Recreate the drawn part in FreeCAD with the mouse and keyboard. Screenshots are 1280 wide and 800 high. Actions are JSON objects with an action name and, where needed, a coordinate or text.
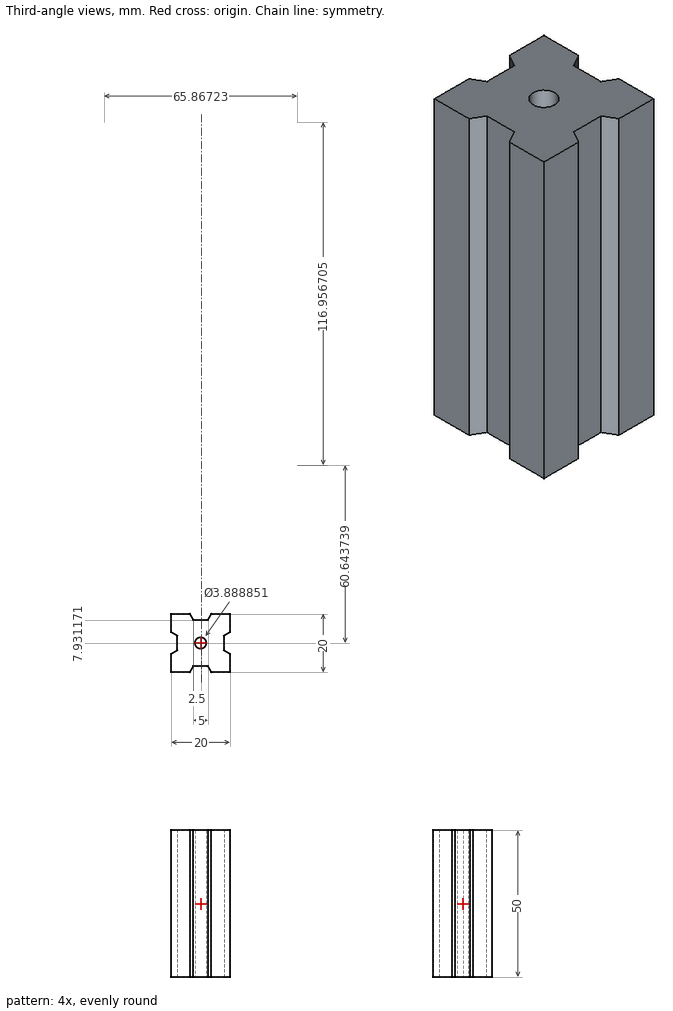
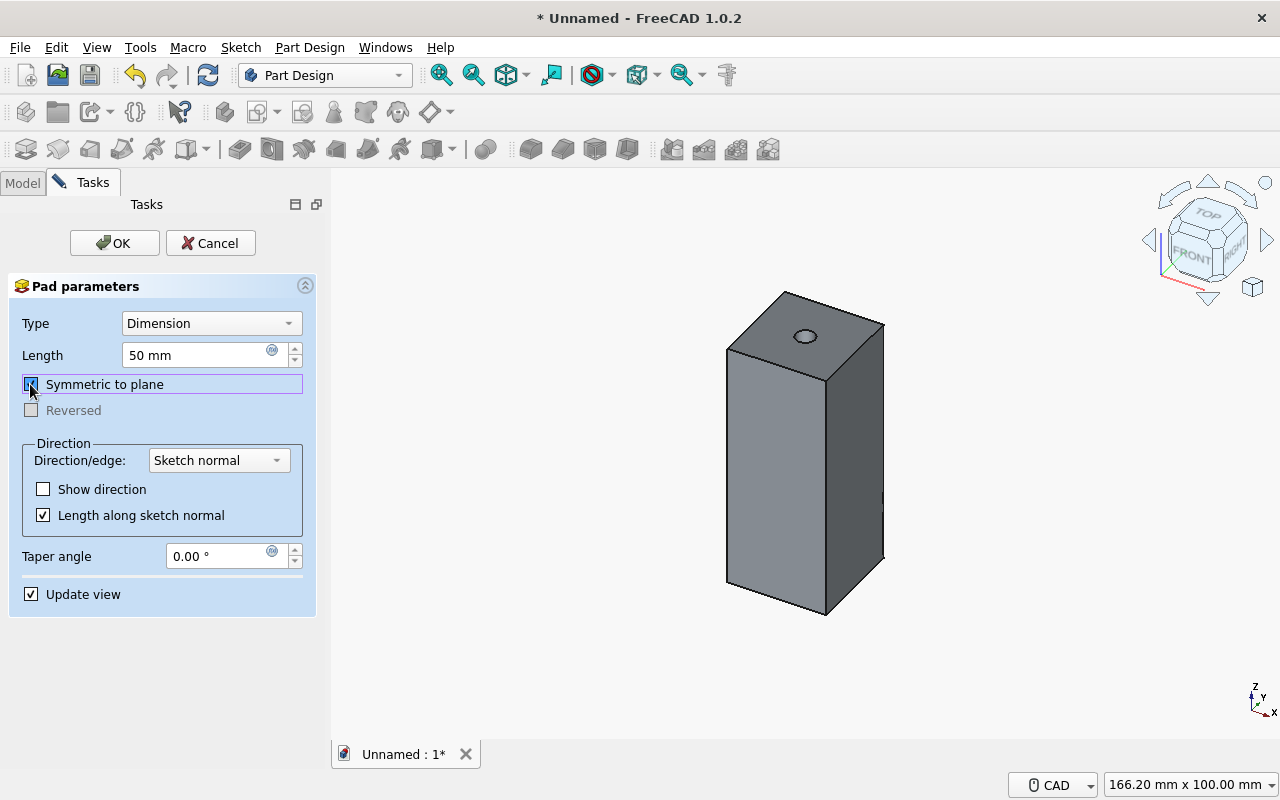
{"action": "left_click", "coordinate": [115, 243]}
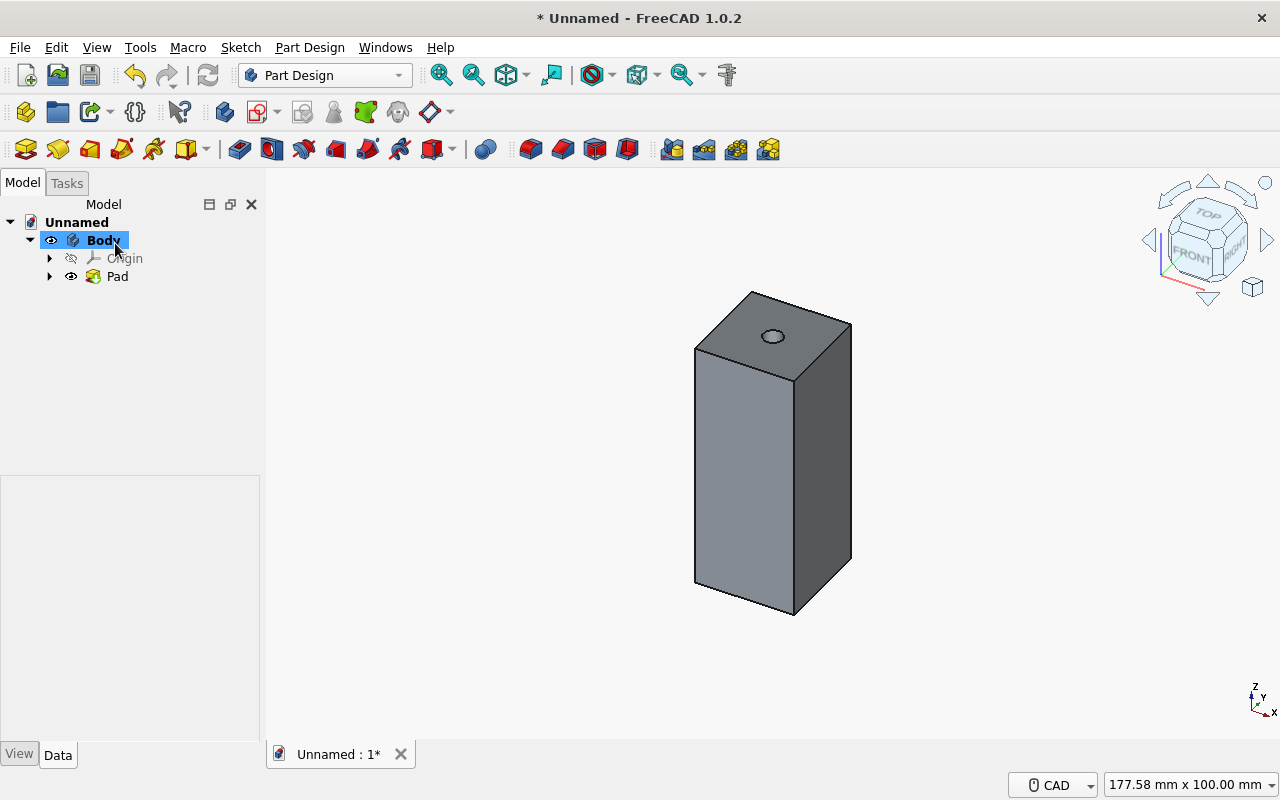
{"action": "left_click", "coordinate": [818, 329]}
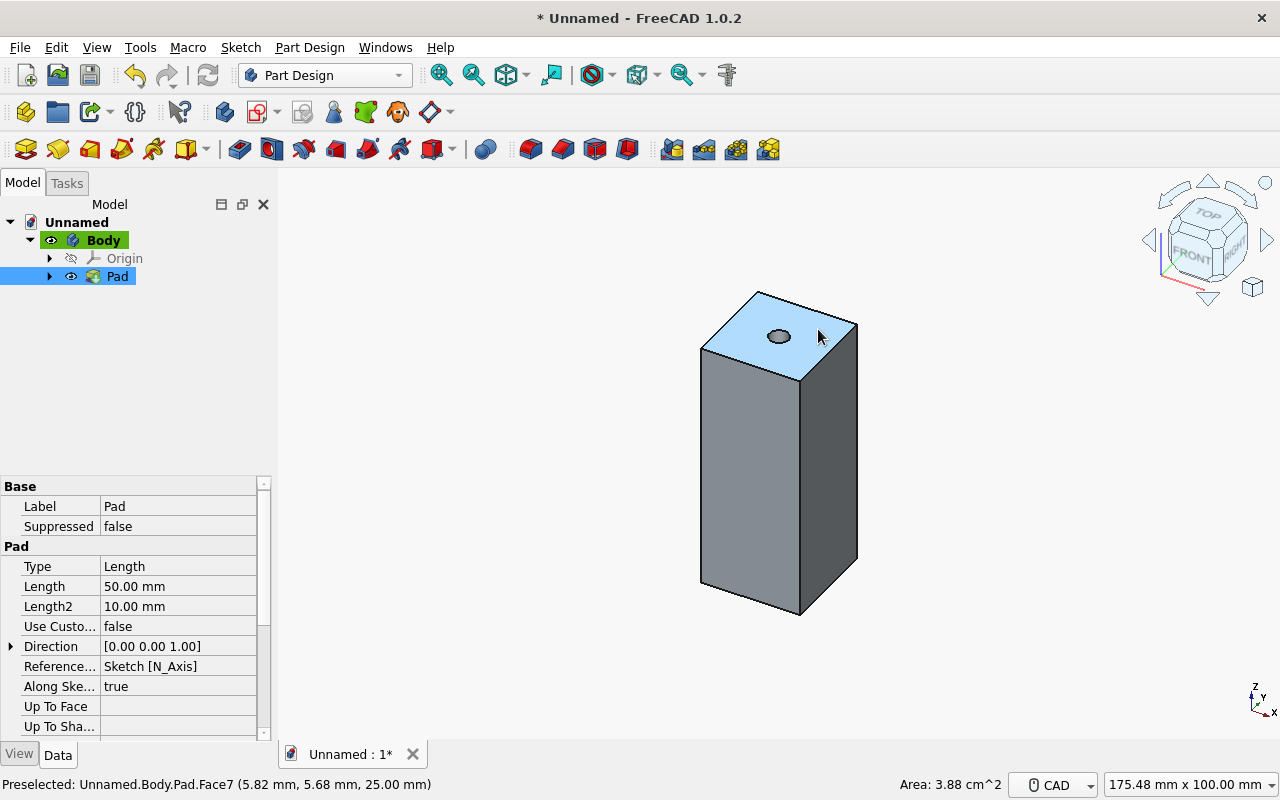
{"action": "left_click", "coordinate": [258, 112]}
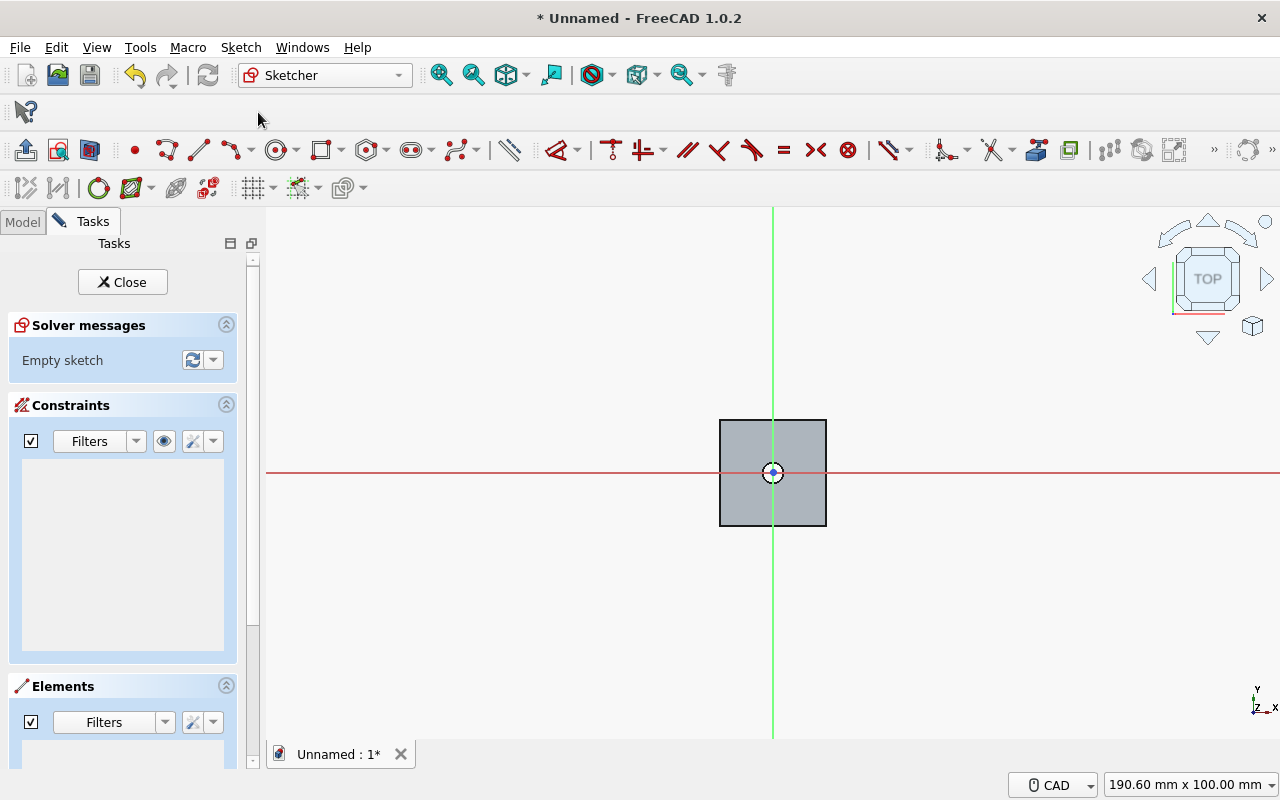
{"action": "scroll", "coordinate": [665, 711], "scroll_direction": "down", "scroll_amount": 5}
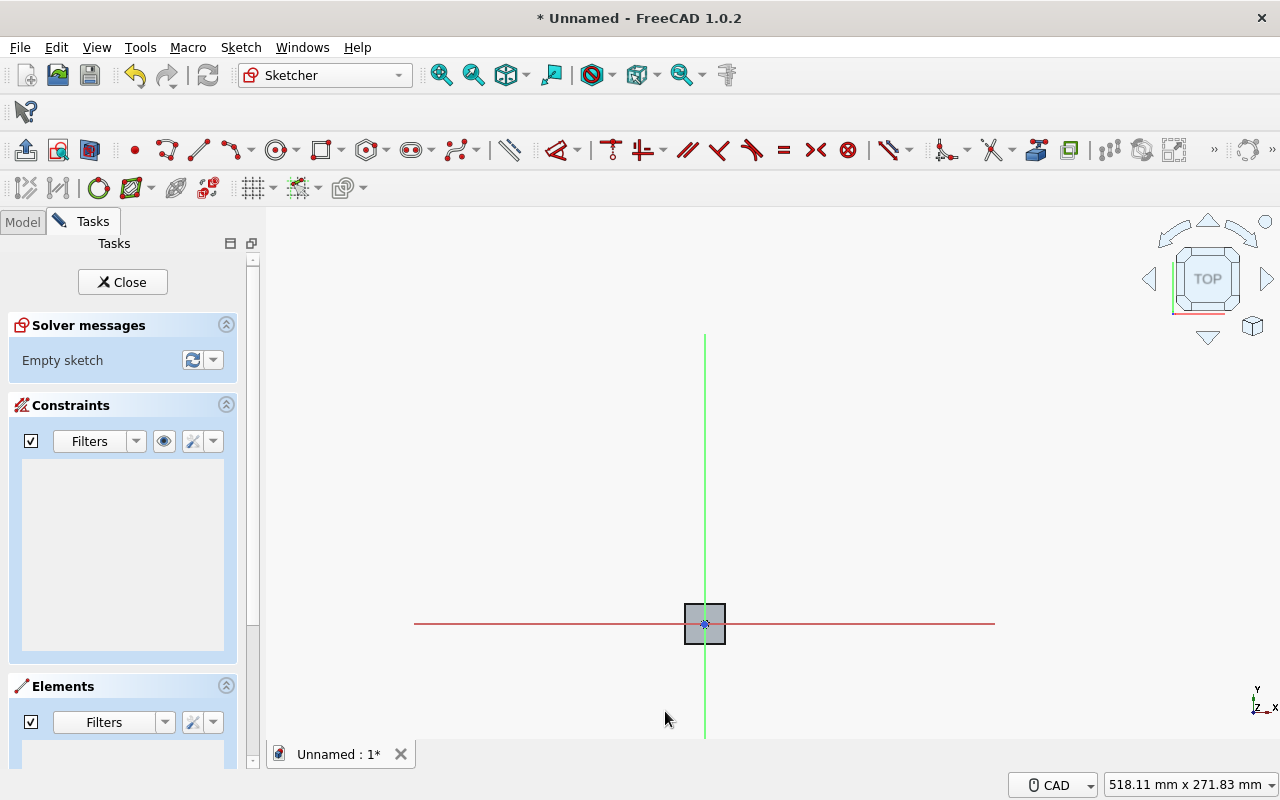
{"action": "left_click", "coordinate": [168, 150]}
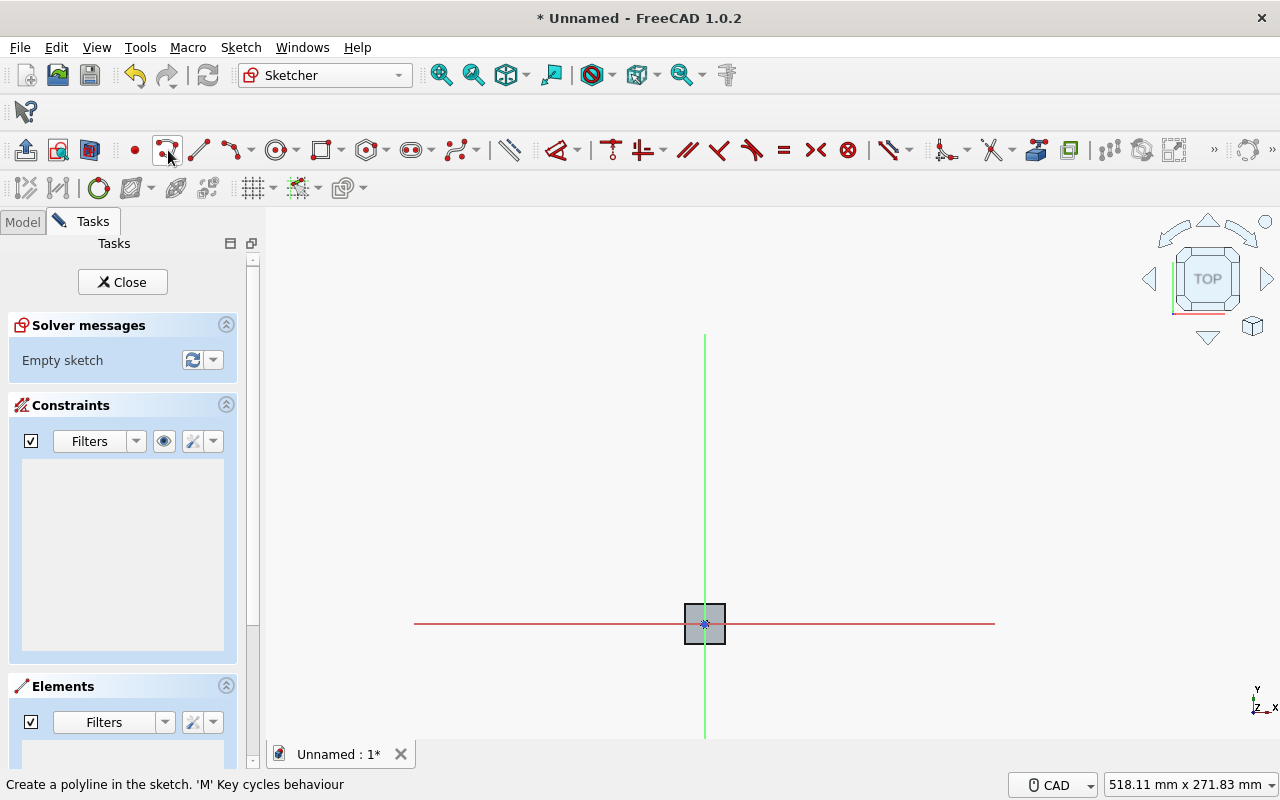
{"action": "scroll", "coordinate": [700, 609], "scroll_direction": "up", "scroll_amount": 6}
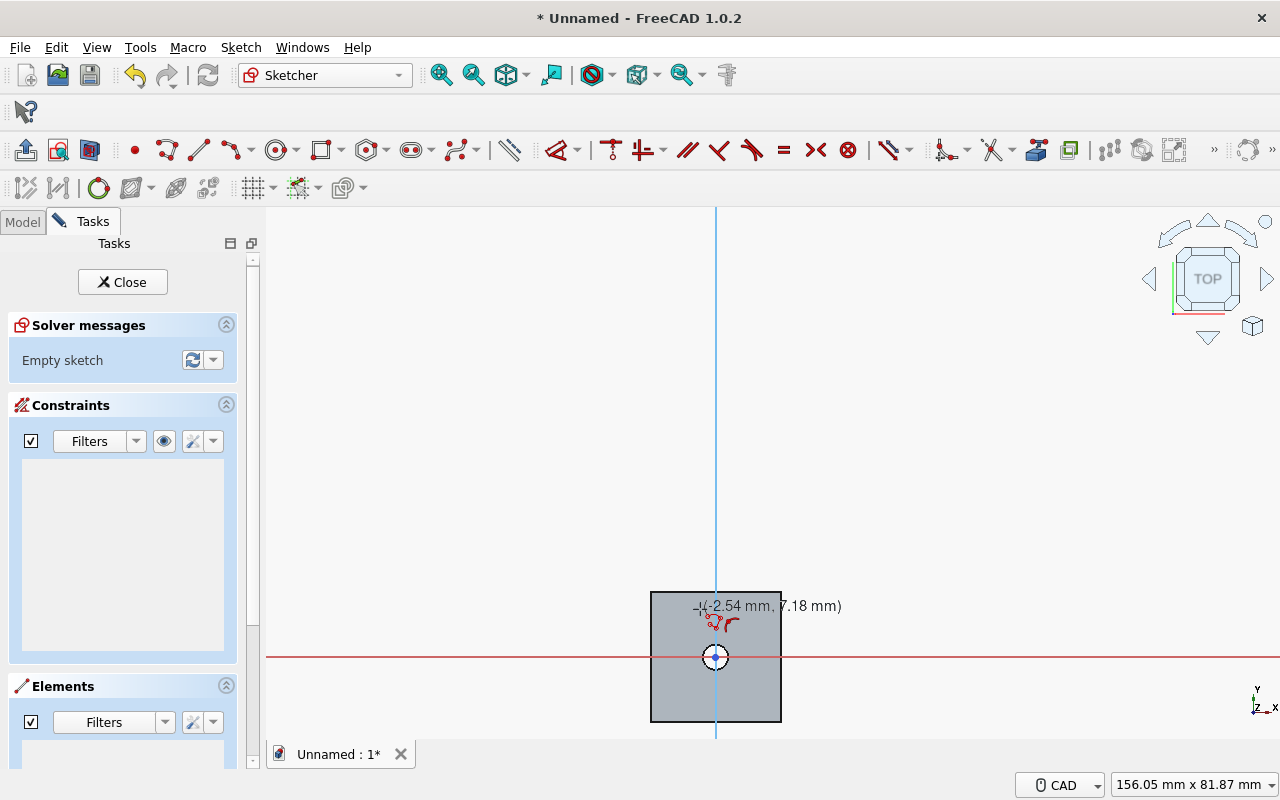
{"action": "left_click", "coordinate": [699, 606]}
{"action": "left_click", "coordinate": [732, 606]}
{"action": "left_click", "coordinate": [930, 263]}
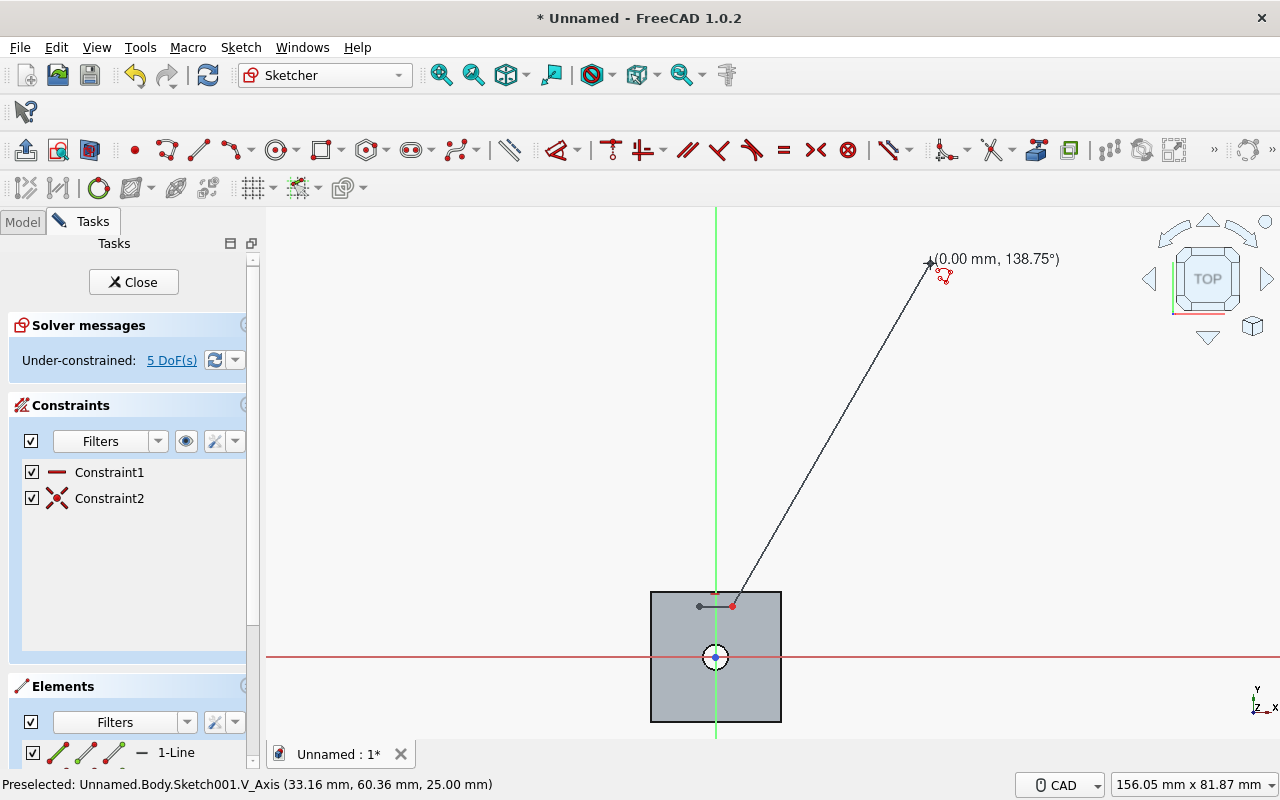
{"action": "scroll", "coordinate": [700, 642], "scroll_direction": "down", "scroll_amount": 6}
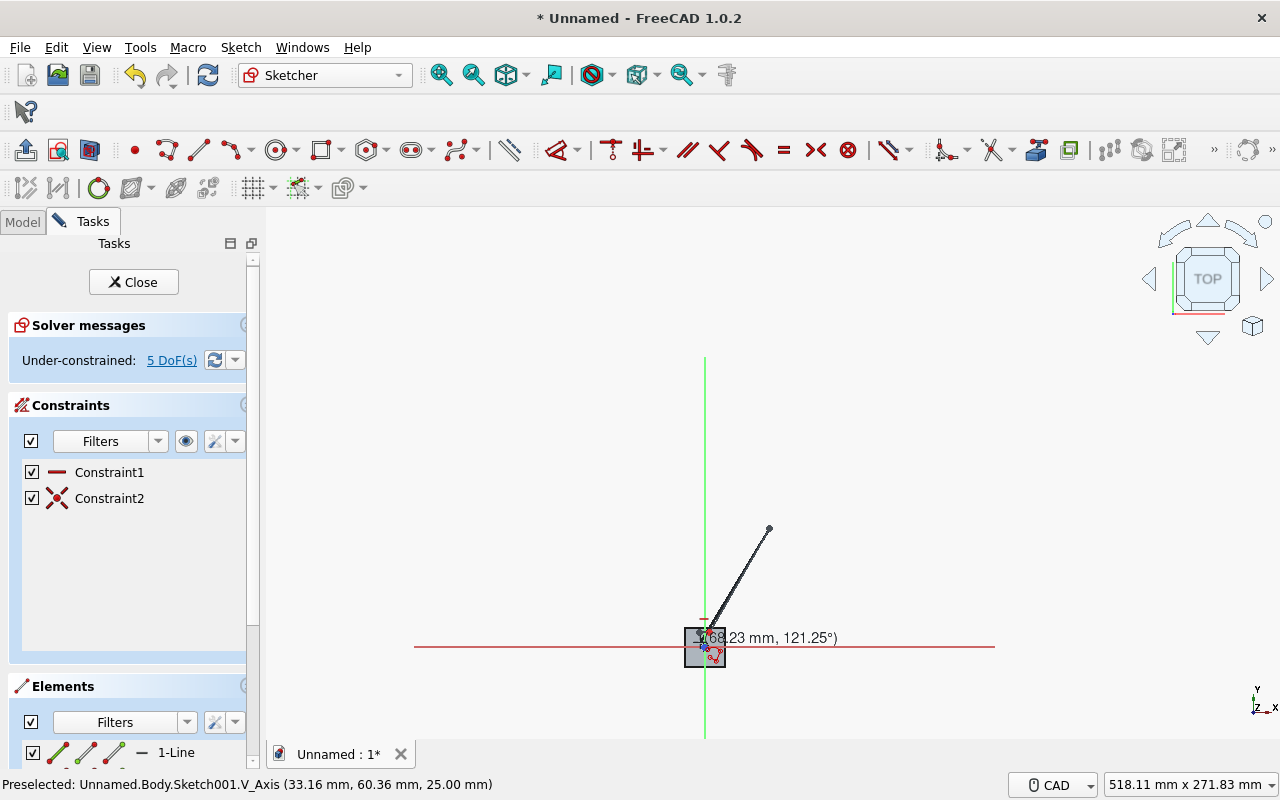
{"action": "left_click", "coordinate": [770, 300]}
{"action": "left_click", "coordinate": [641, 300]}
{"action": "left_click", "coordinate": [641, 528]}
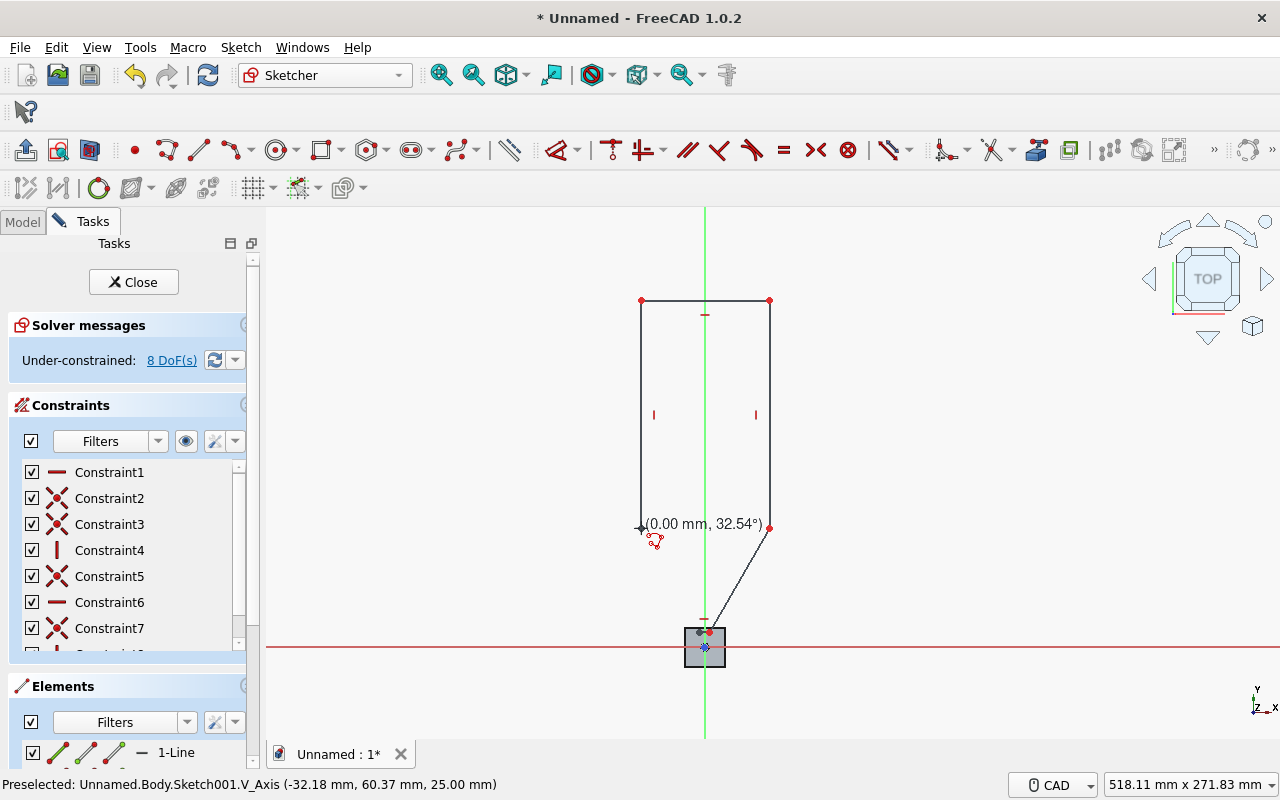
{"action": "scroll", "coordinate": [700, 632], "scroll_direction": "up", "scroll_amount": 6}